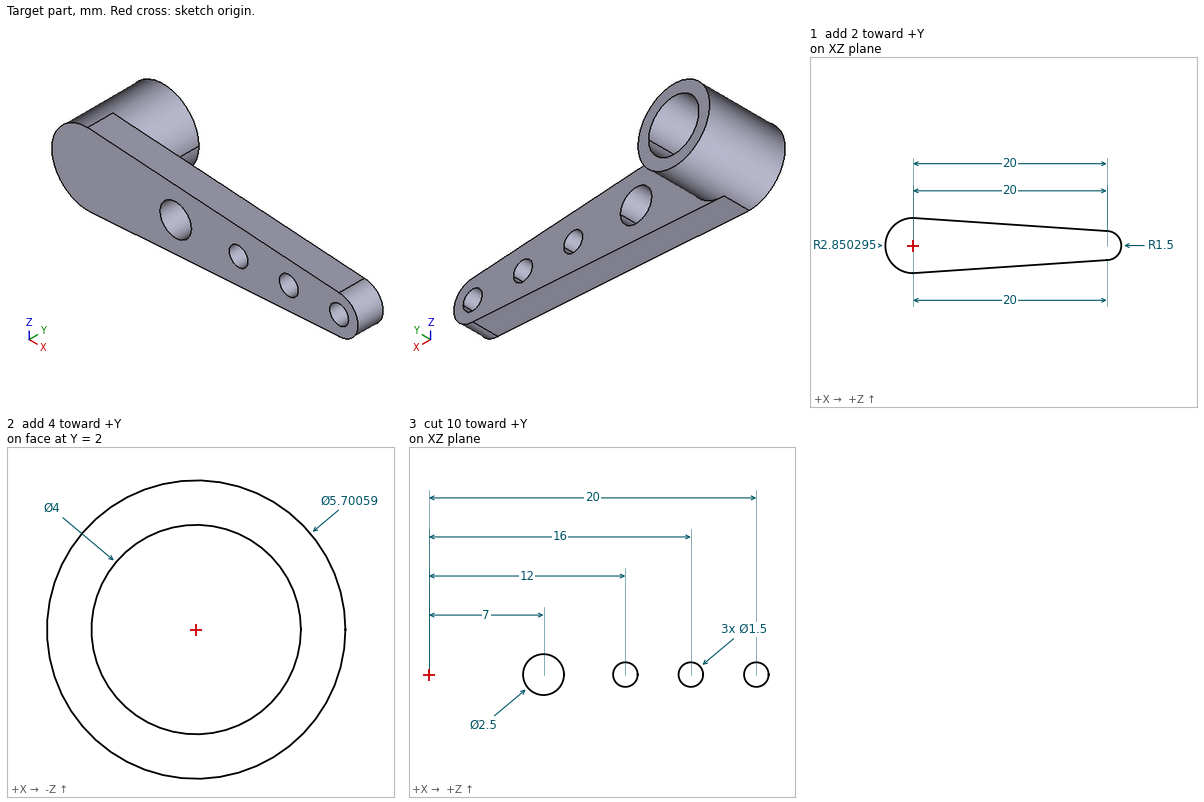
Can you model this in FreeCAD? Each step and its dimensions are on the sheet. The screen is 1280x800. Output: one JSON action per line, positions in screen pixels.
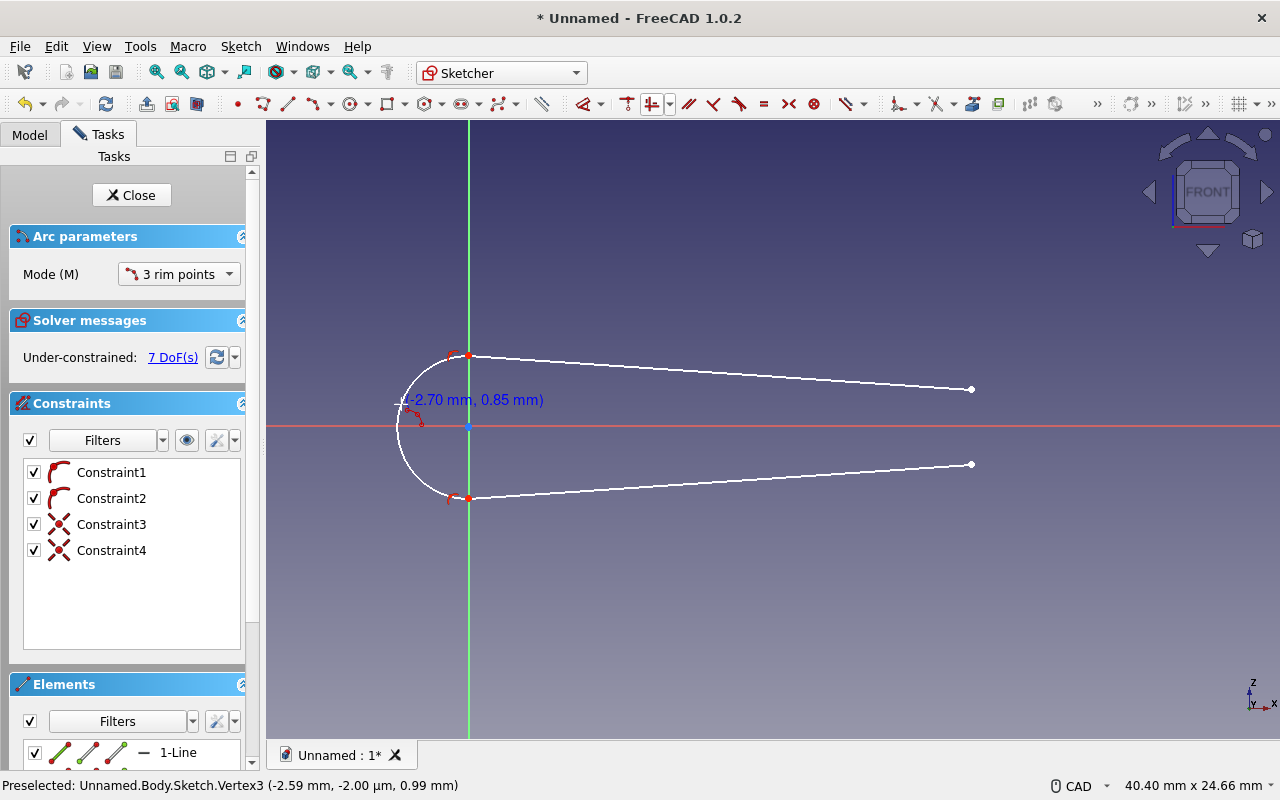
{"action": "left_click", "coordinate": [971, 390]}
{"action": "left_click", "coordinate": [971, 465]}
{"action": "left_click", "coordinate": [1001, 449]}
{"action": "key", "text": "Escape"}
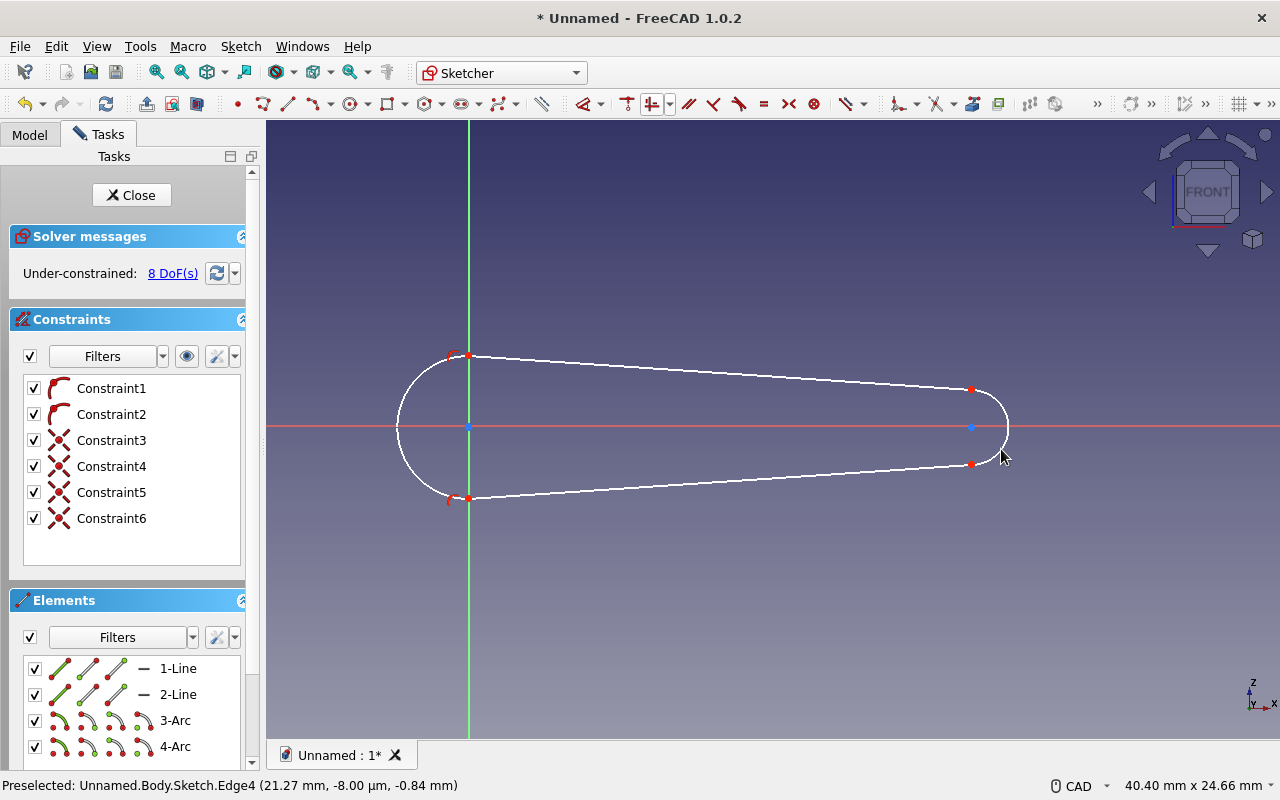
{"action": "left_click_drag", "start_coordinate": [459, 416], "coordinate": [479, 438]}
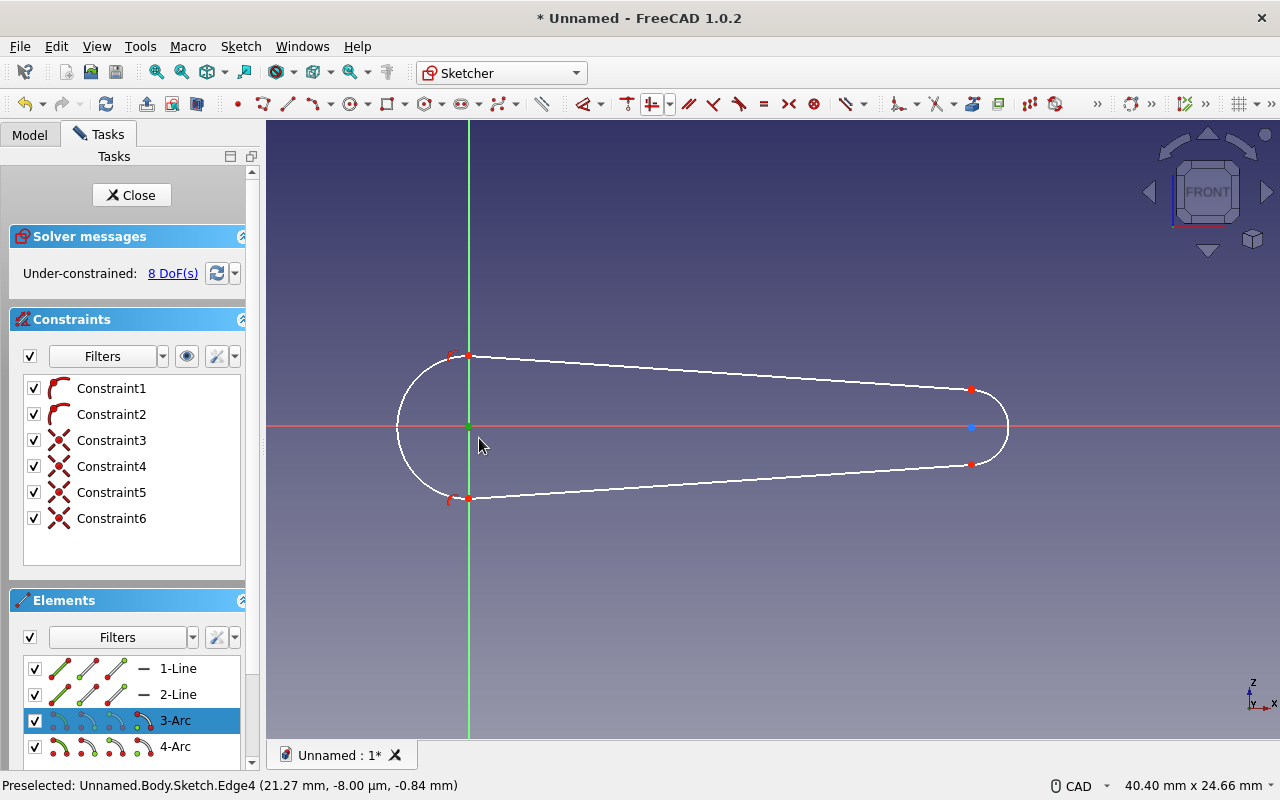
{"action": "left_click", "coordinate": [627, 104]}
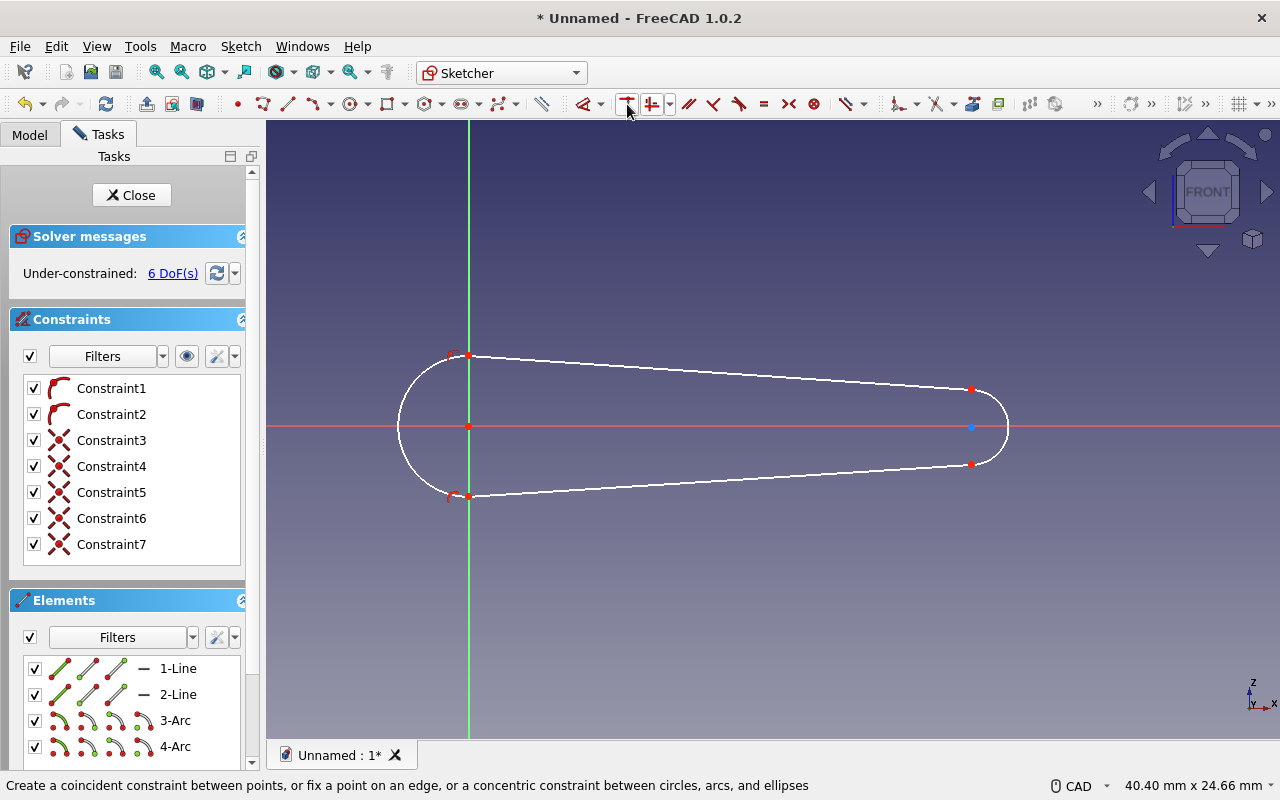
{"action": "left_click", "coordinate": [971, 427]}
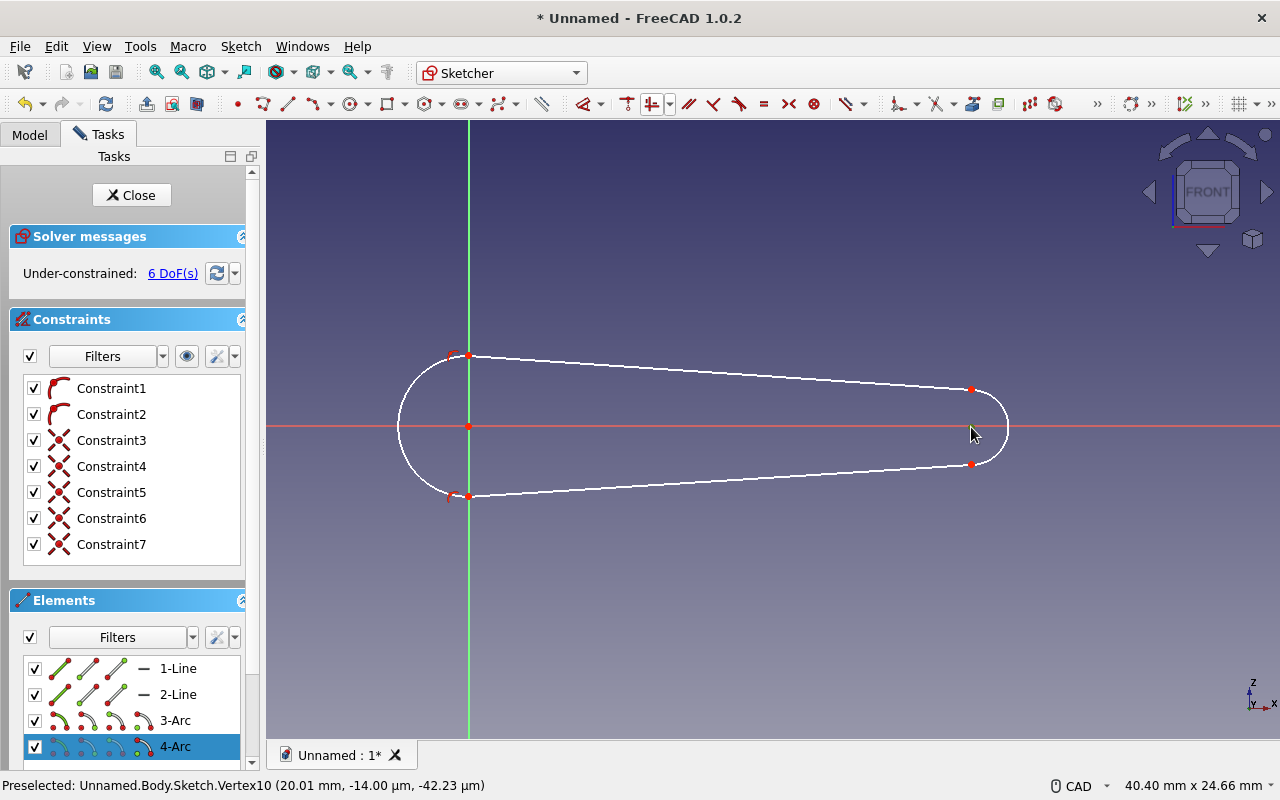
{"action": "left_click", "coordinate": [353, 426]}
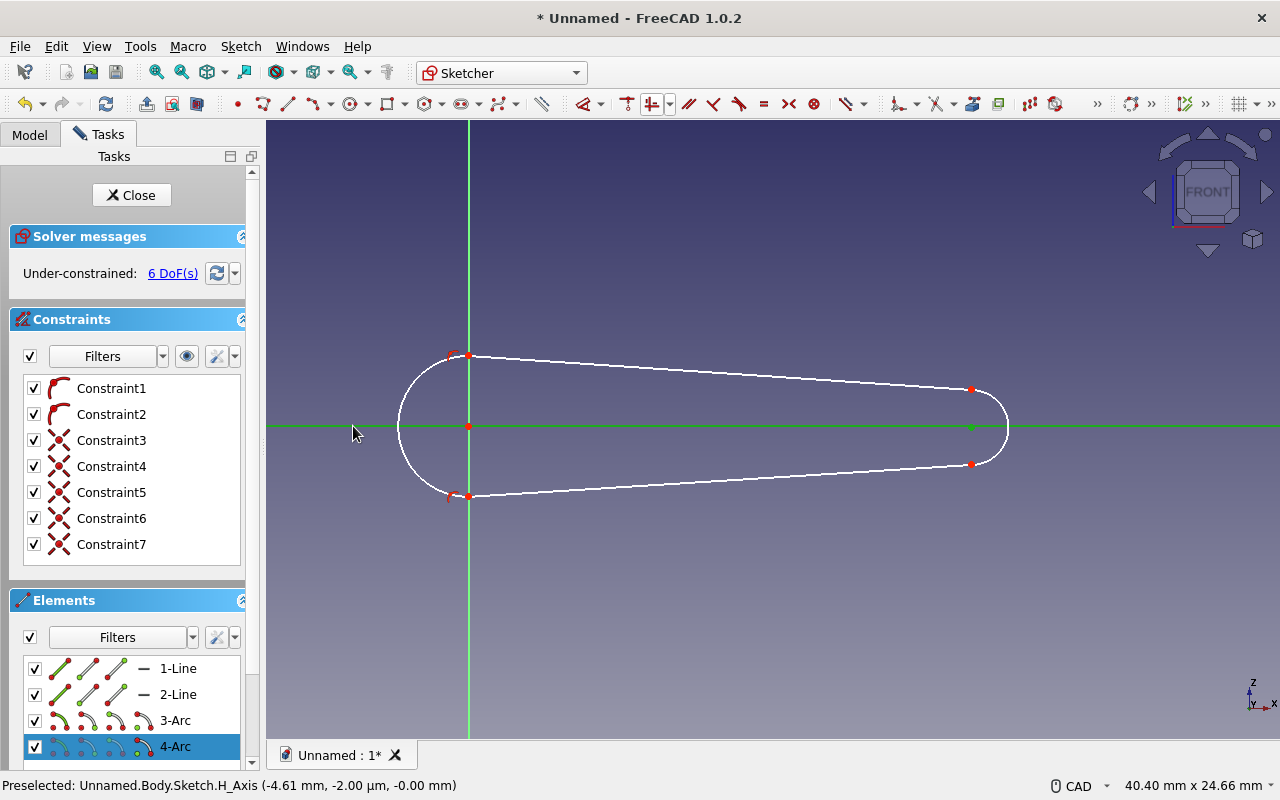
{"action": "left_click", "coordinate": [627, 104]}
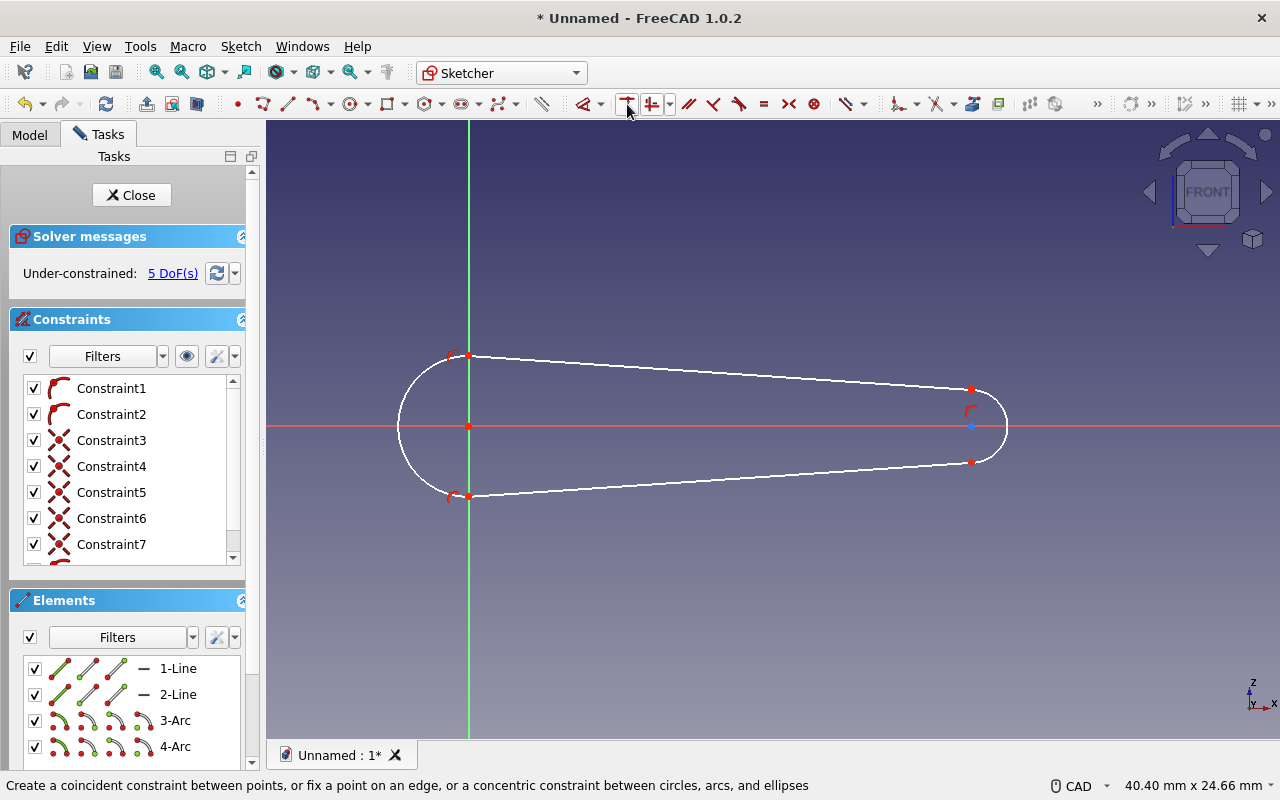
{"action": "left_click", "coordinate": [582, 104]}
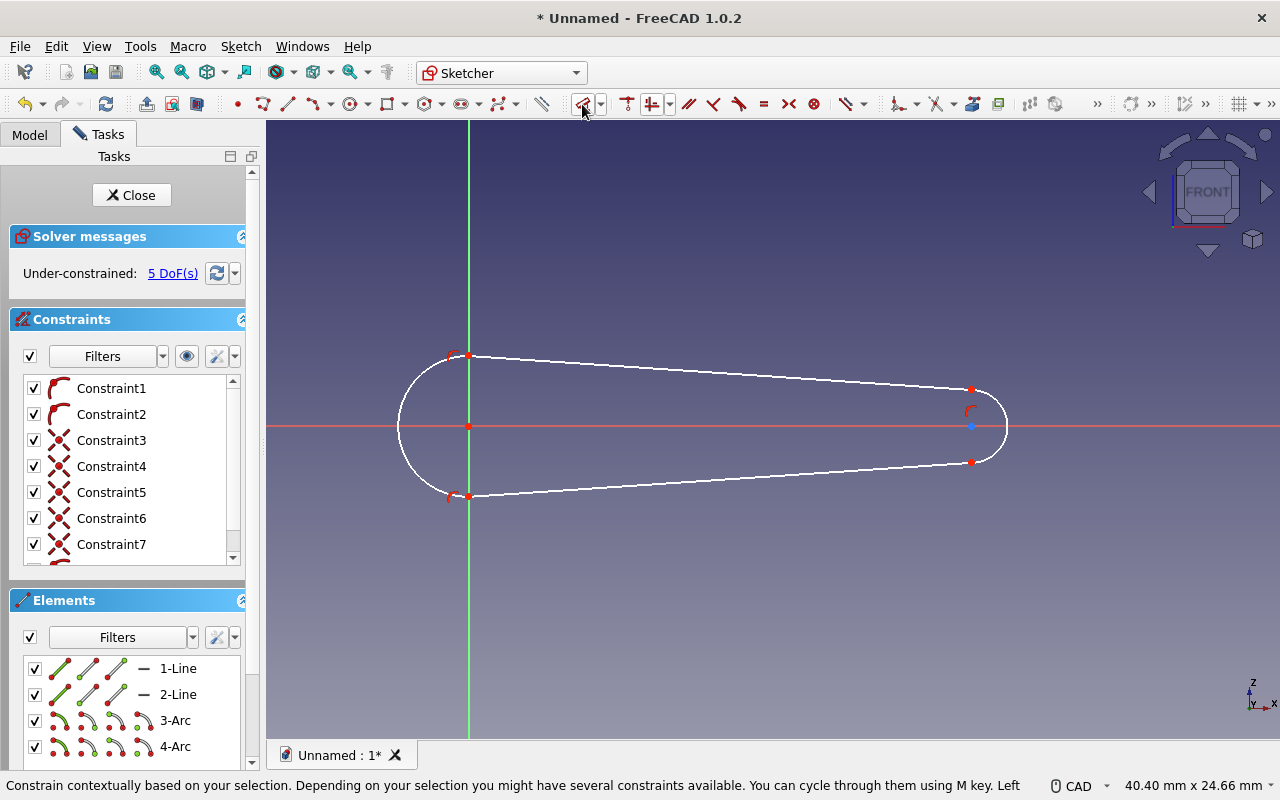
{"action": "left_click", "coordinate": [412, 385]}
{"action": "left_click", "coordinate": [386, 366]}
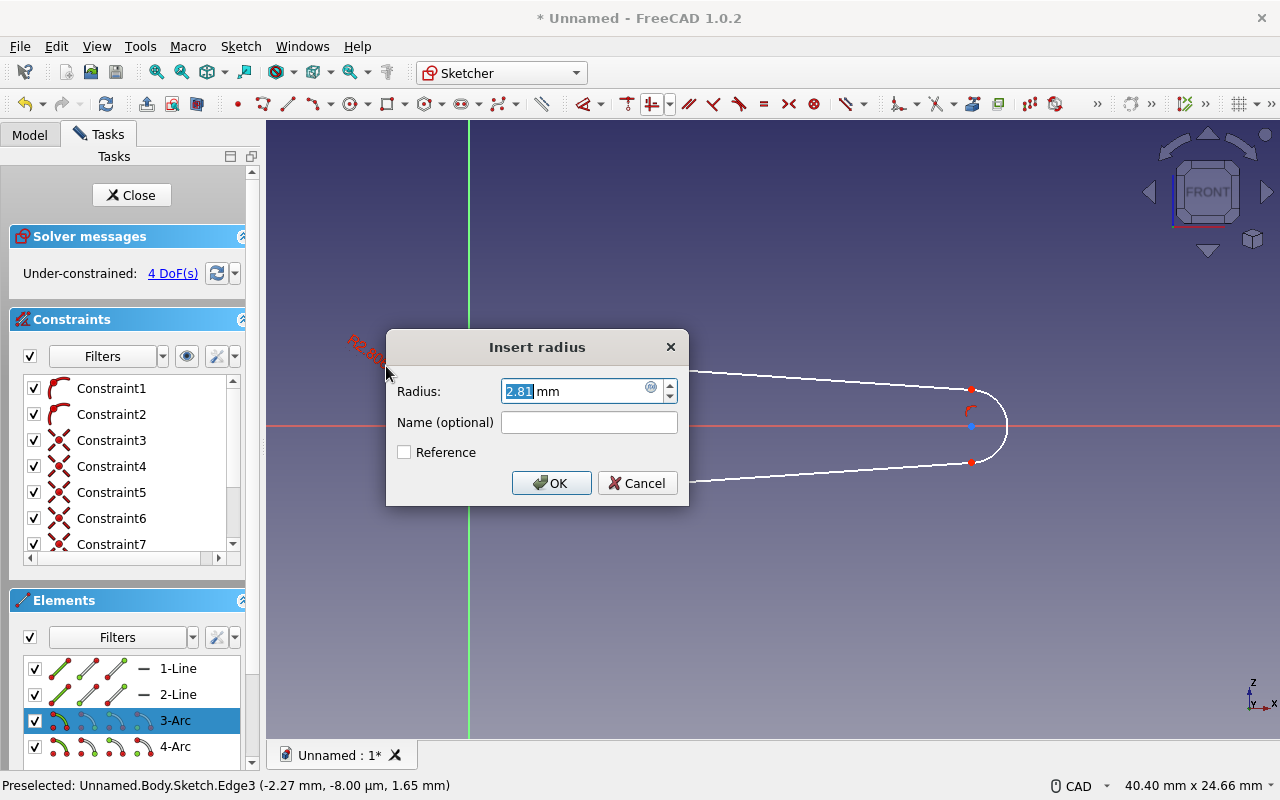
{"action": "type", "text": "2.850295"}
{"action": "key", "text": "Return"}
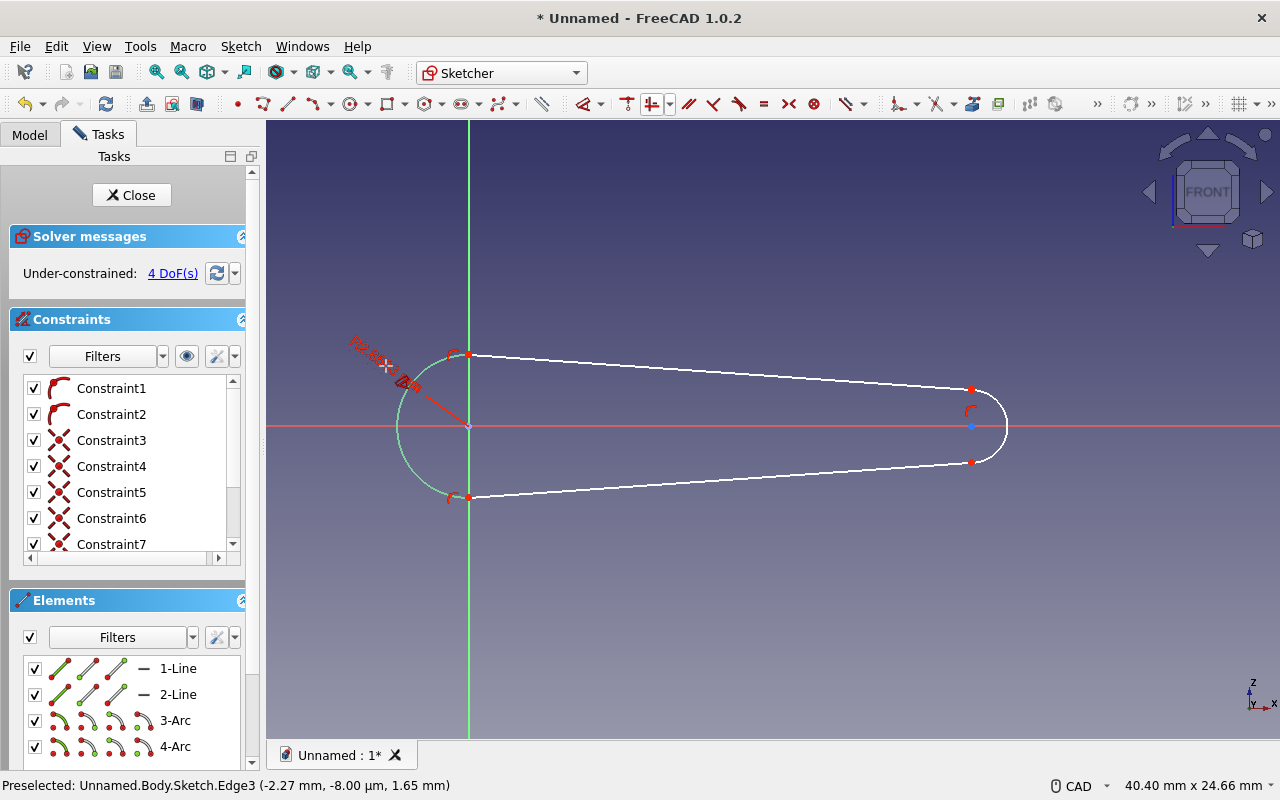
{"action": "left_click", "coordinate": [1000, 448]}
{"action": "left_click", "coordinate": [1026, 467]}